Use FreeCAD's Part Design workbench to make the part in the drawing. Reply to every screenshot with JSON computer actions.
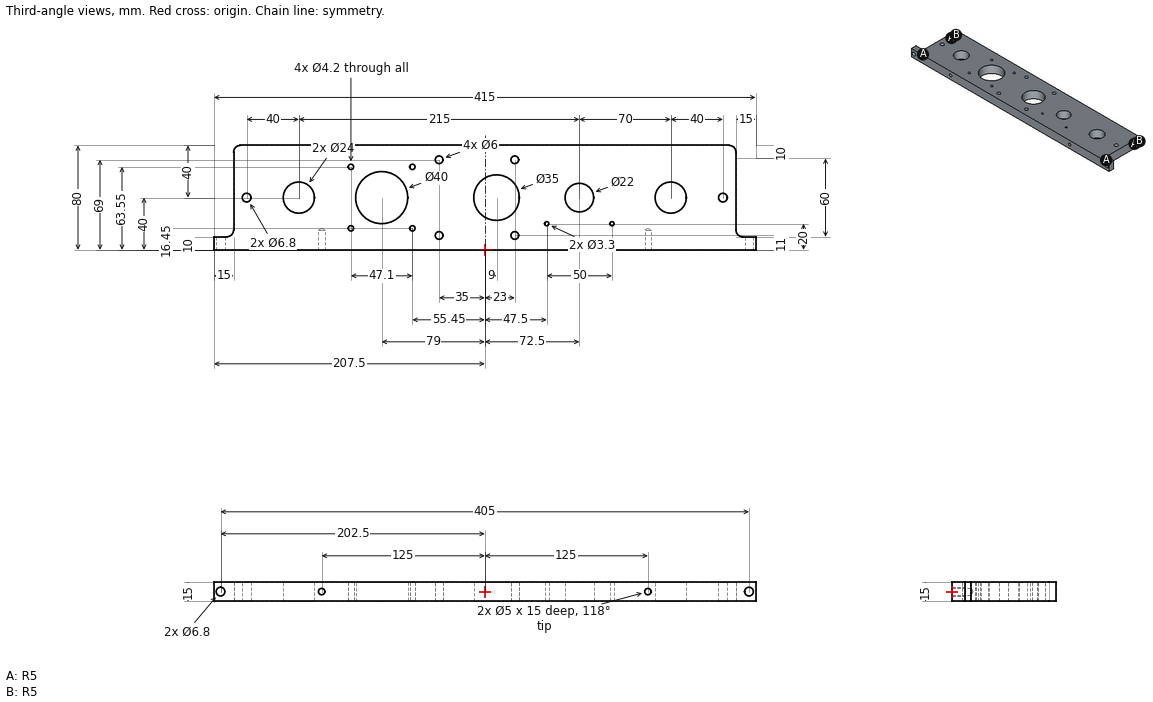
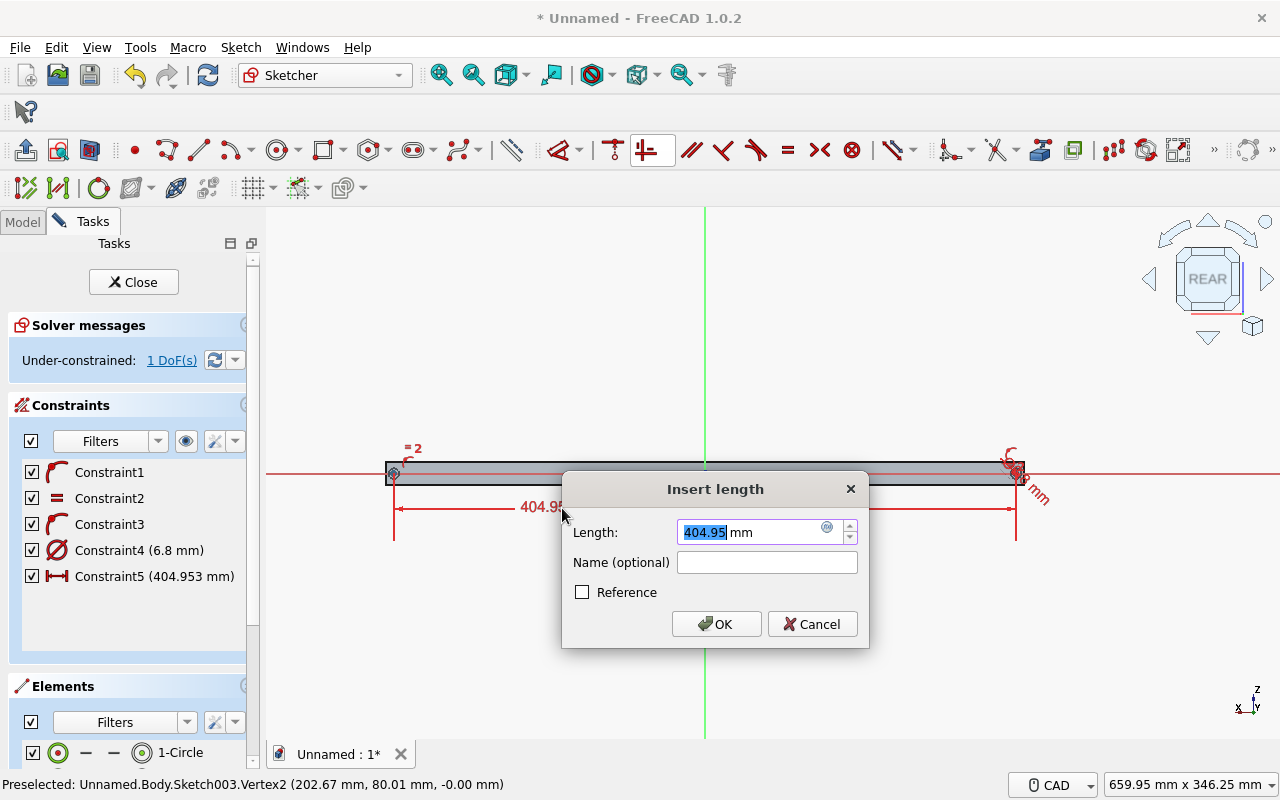
{"action": "type", "text": "405"}
{"action": "key", "text": "Return"}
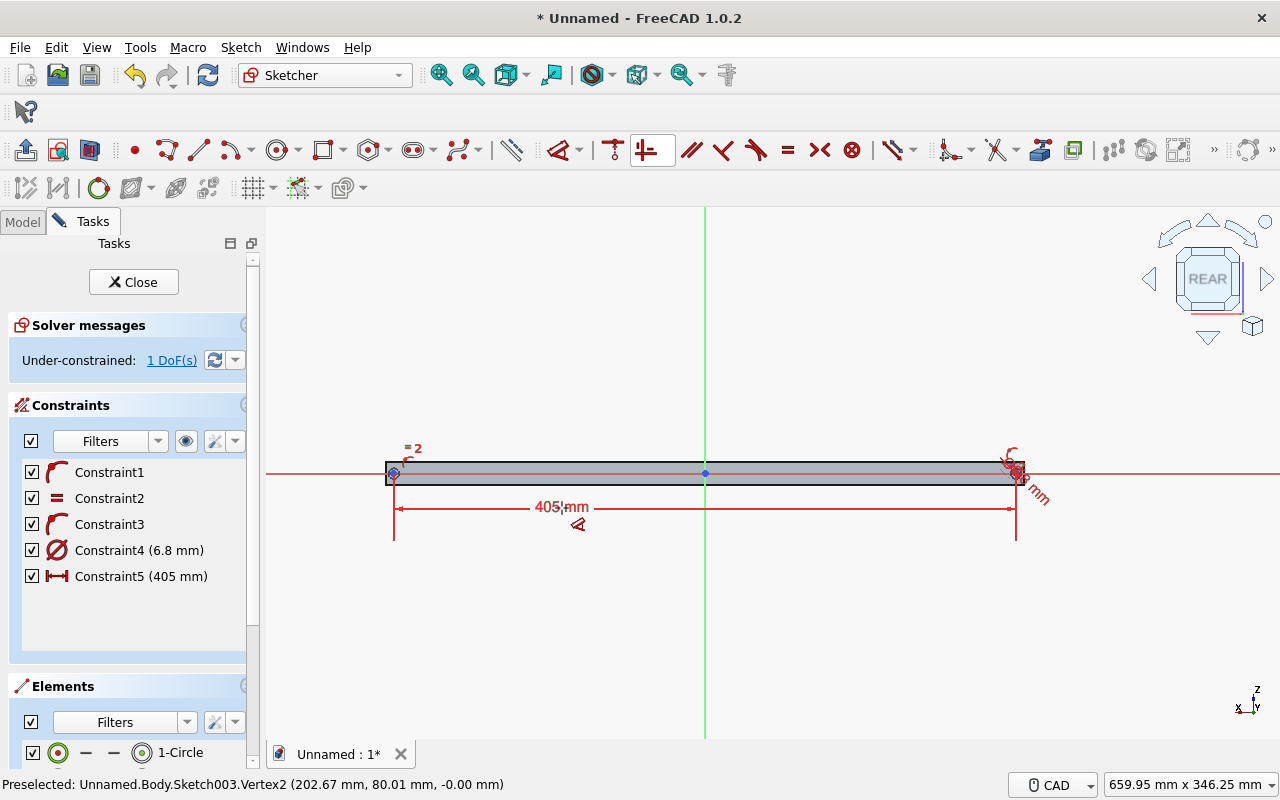
{"action": "left_click", "coordinate": [1016, 474]}
{"action": "left_click", "coordinate": [861, 508]}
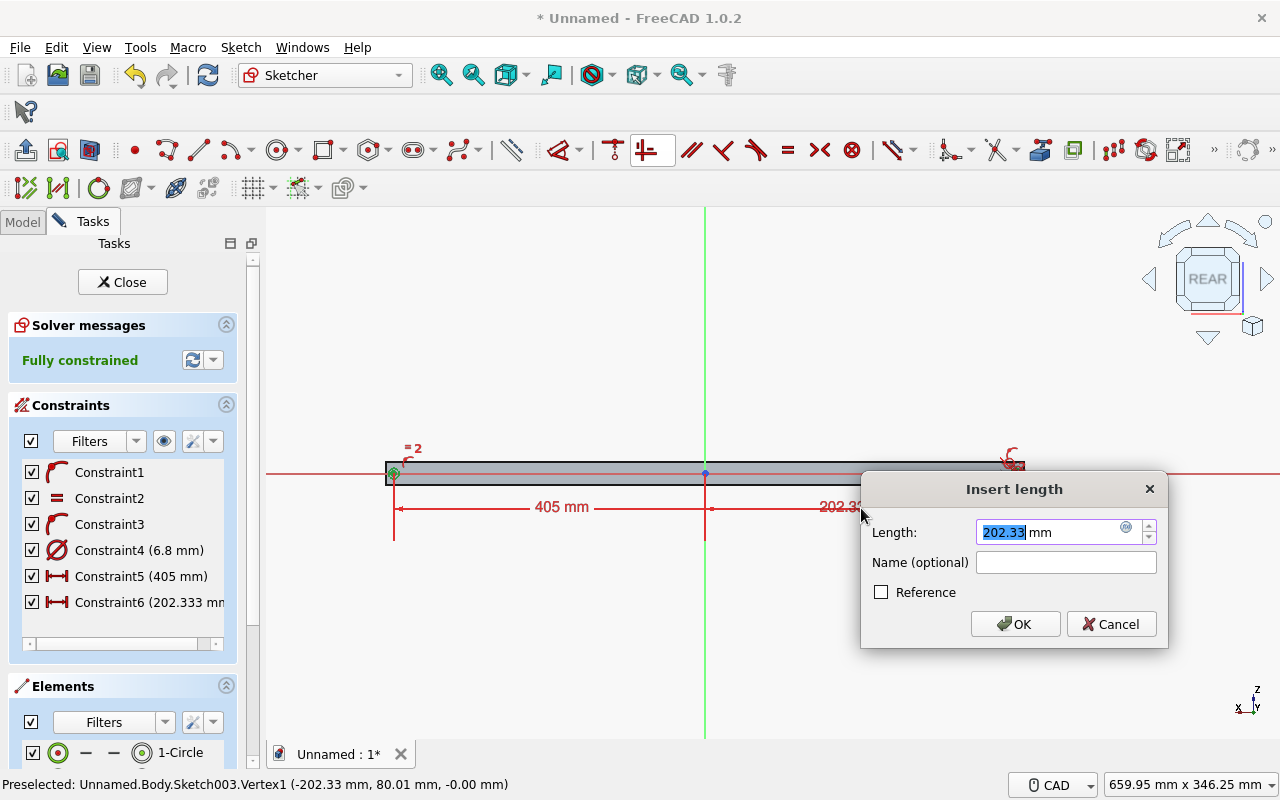
{"action": "type", "text": "202.5"}
{"action": "key", "text": "Return"}
{"action": "key", "text": "Escape"}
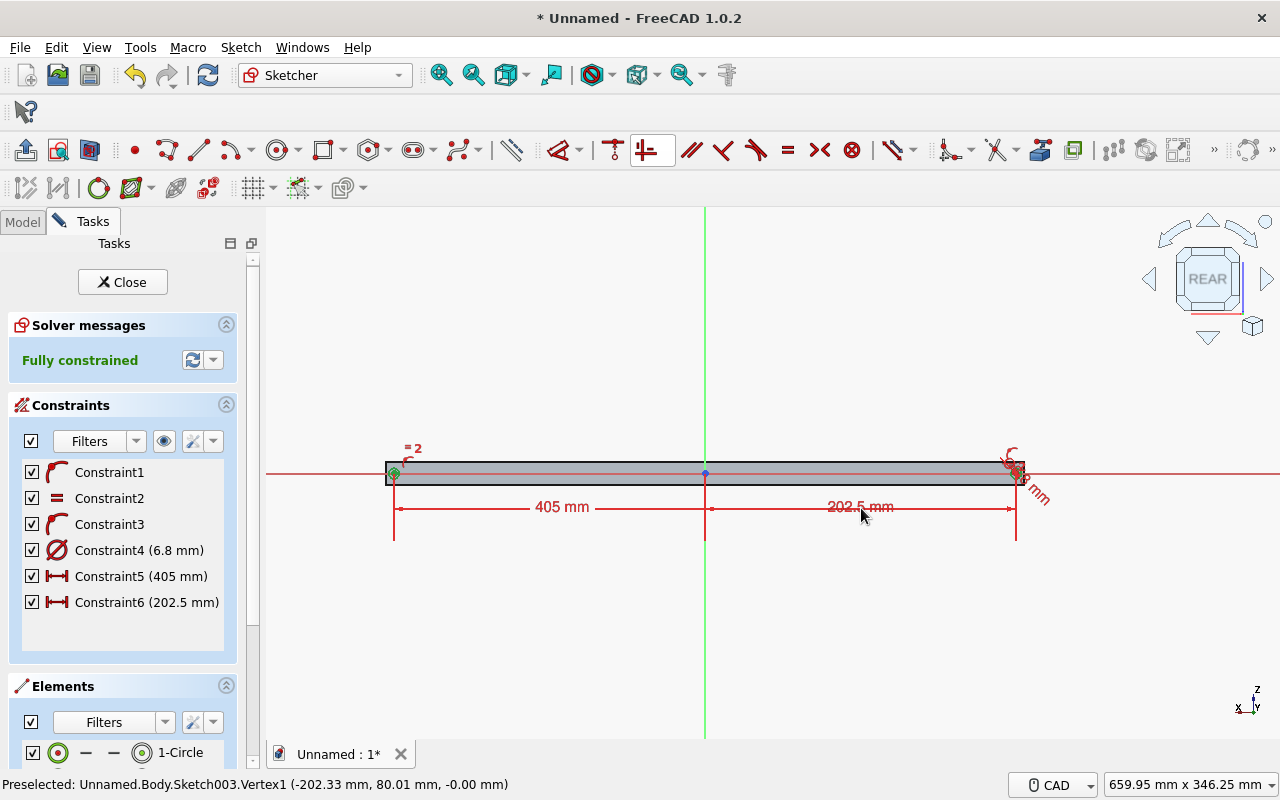
{"action": "left_click", "coordinate": [123, 282]}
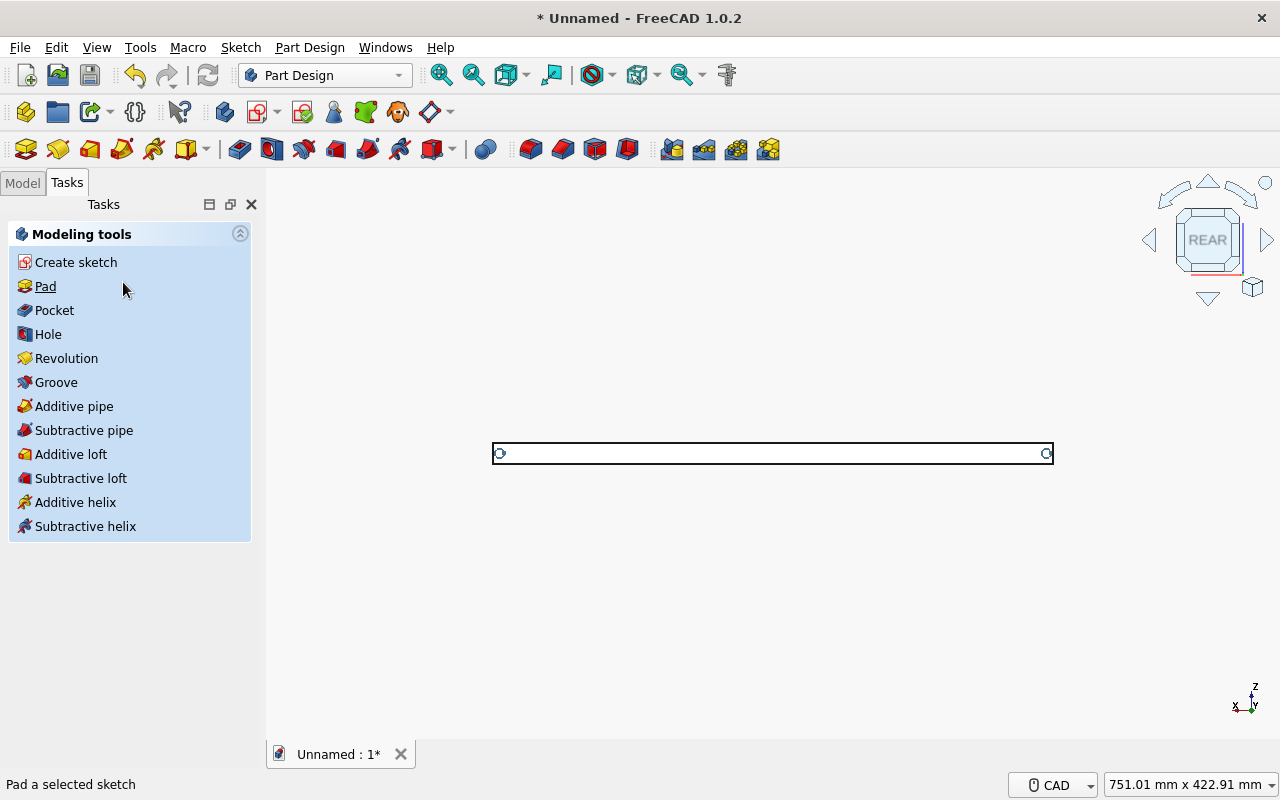
{"action": "left_click", "coordinate": [240, 150]}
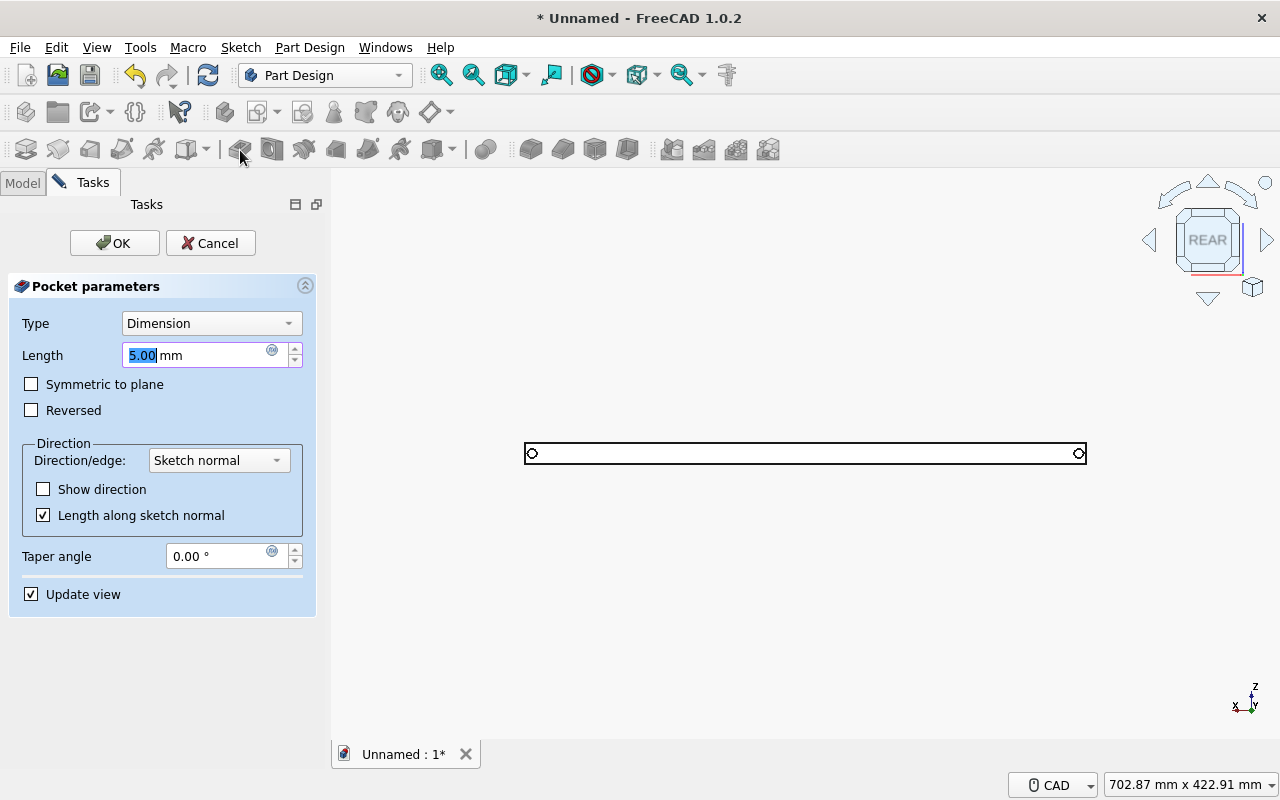
{"action": "left_click", "coordinate": [212, 324]}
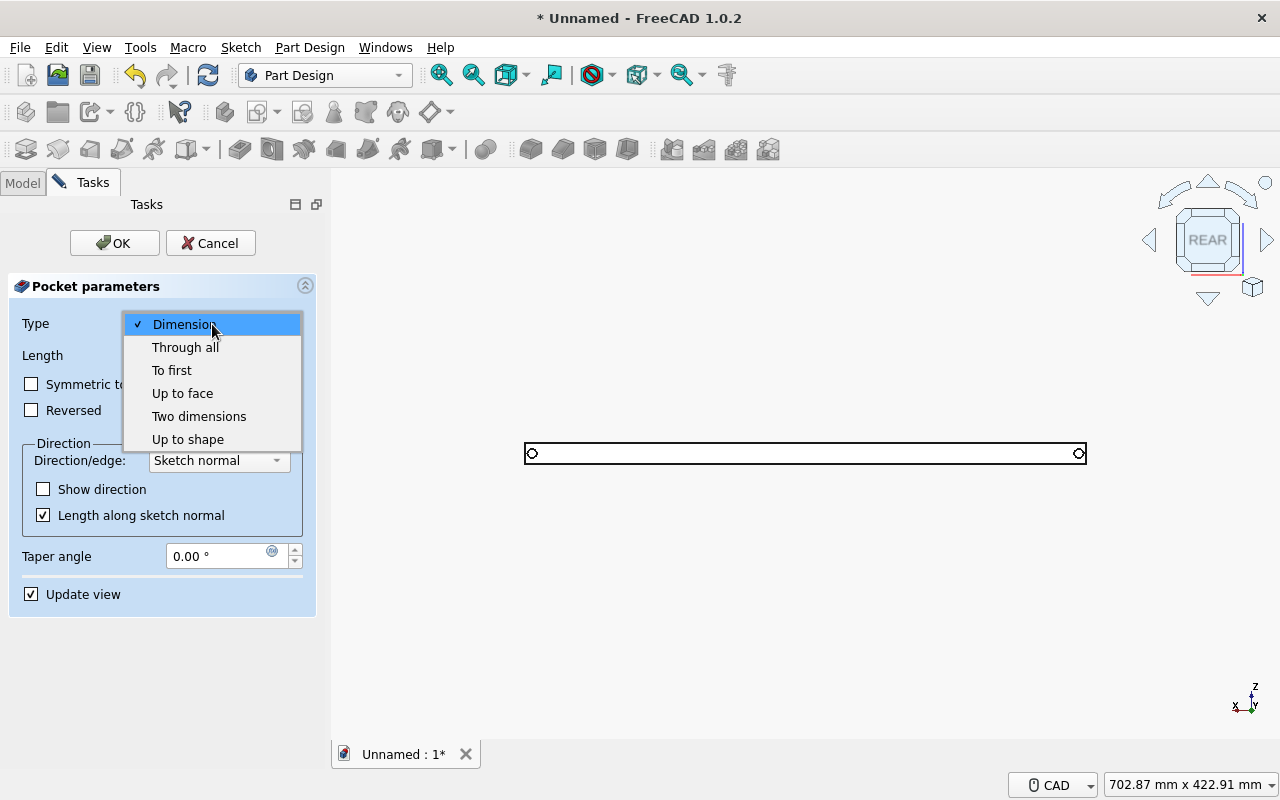
{"action": "left_click", "coordinate": [212, 348]}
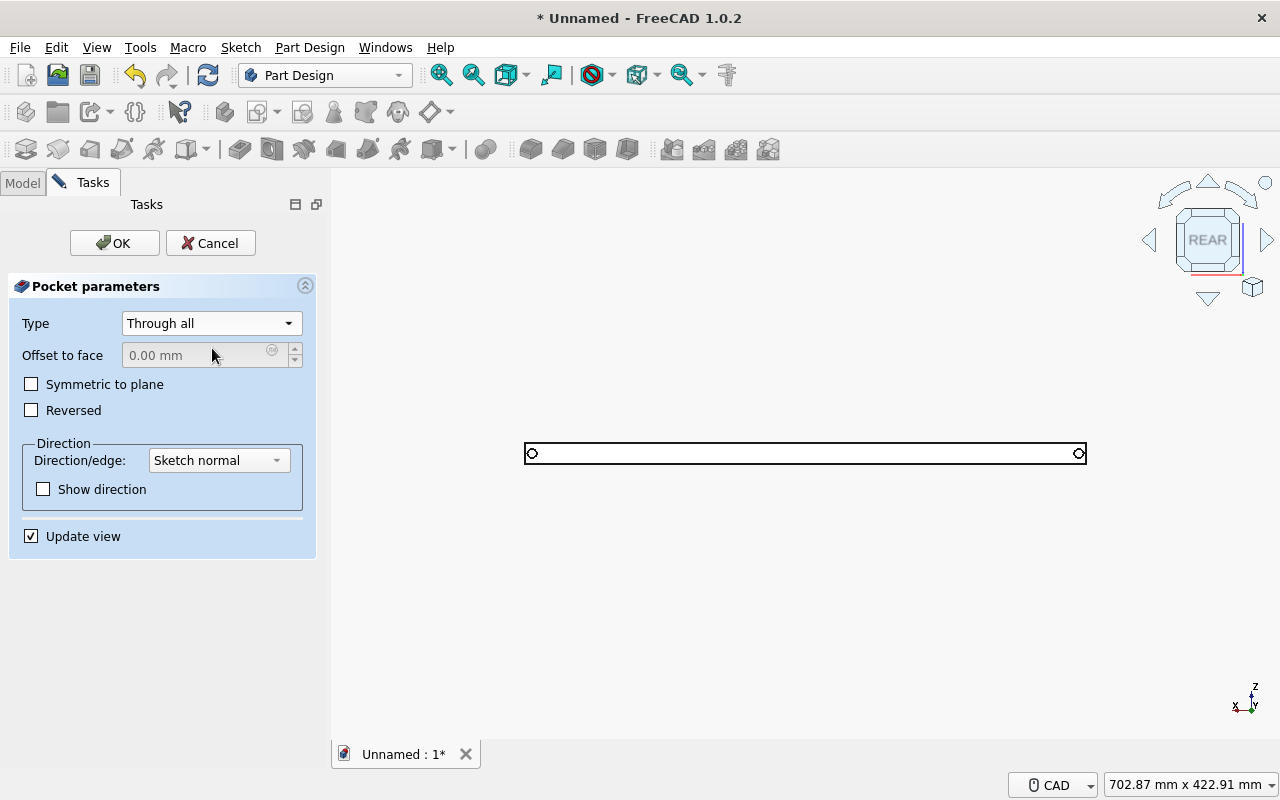
{"action": "left_click", "coordinate": [115, 243]}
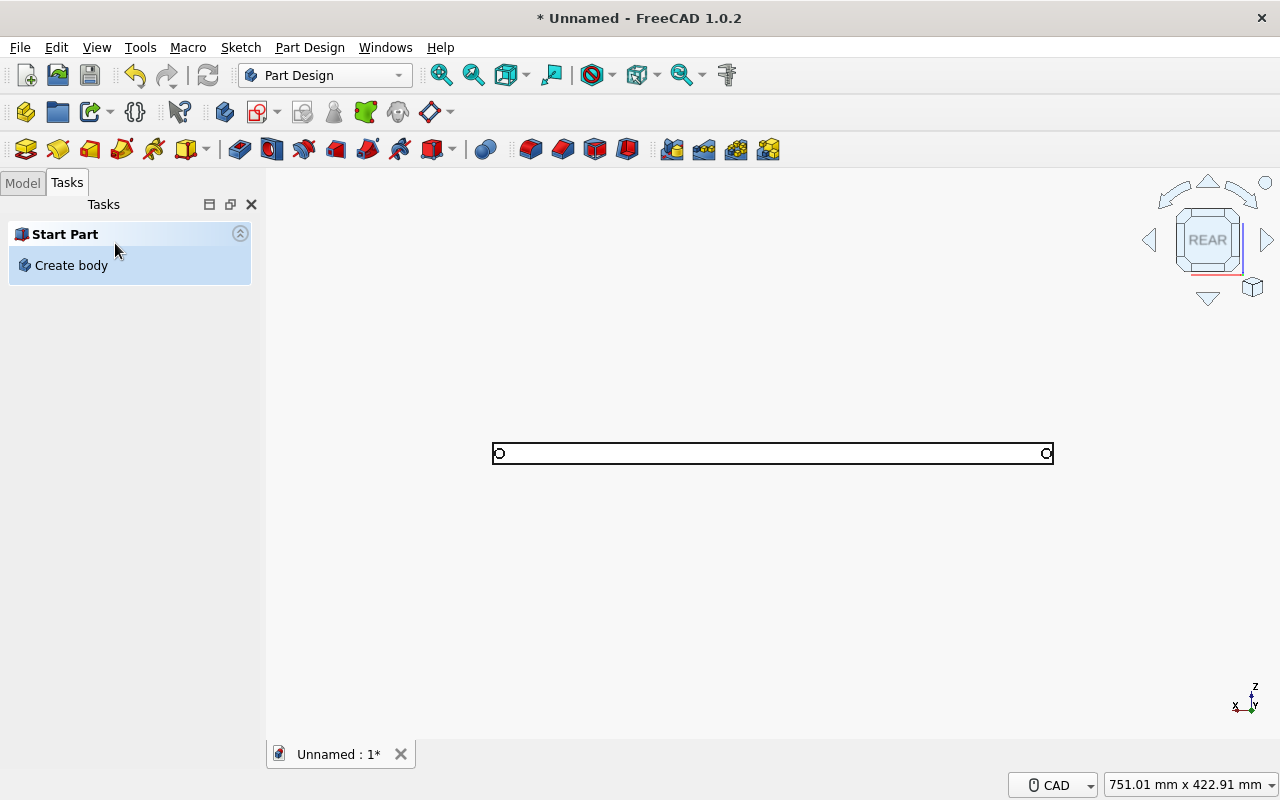
{"action": "scroll", "coordinate": [1033, 453], "scroll_direction": "up", "scroll_amount": 4}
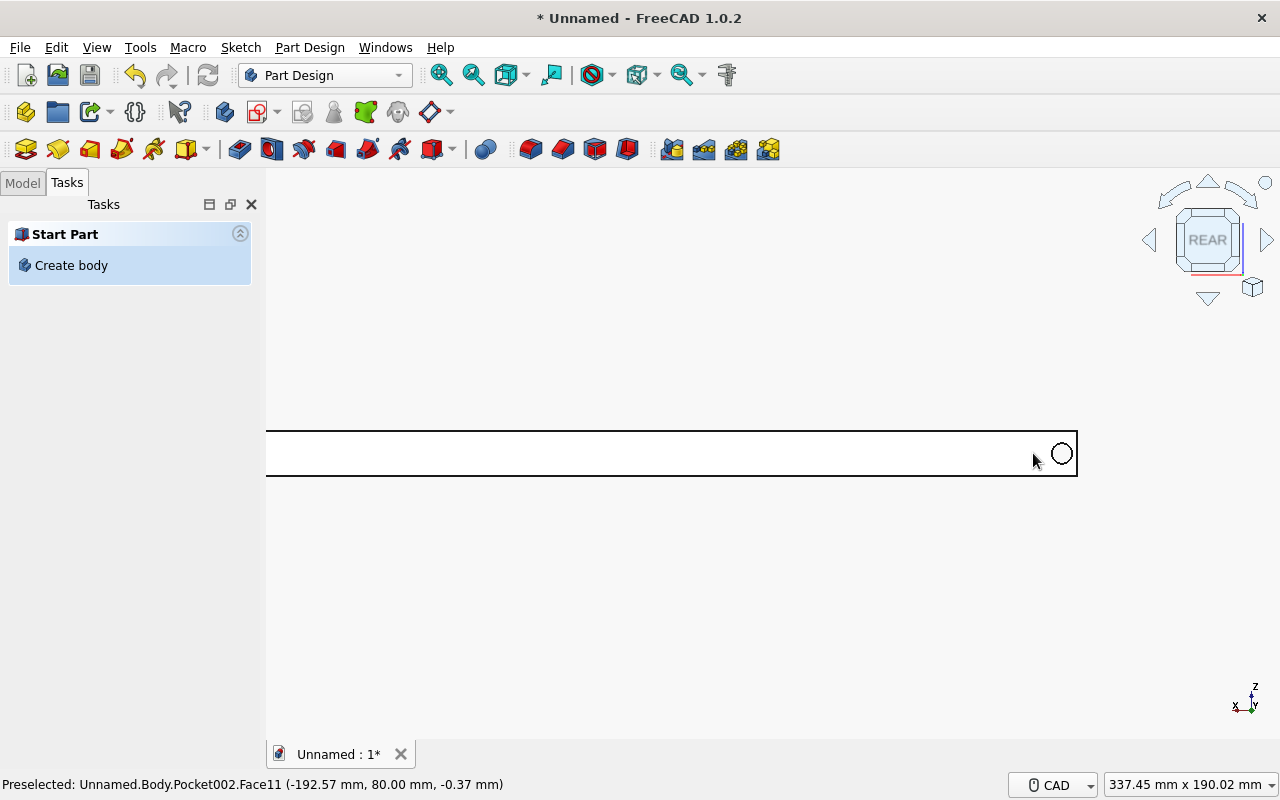
{"action": "left_click", "coordinate": [442, 76]}